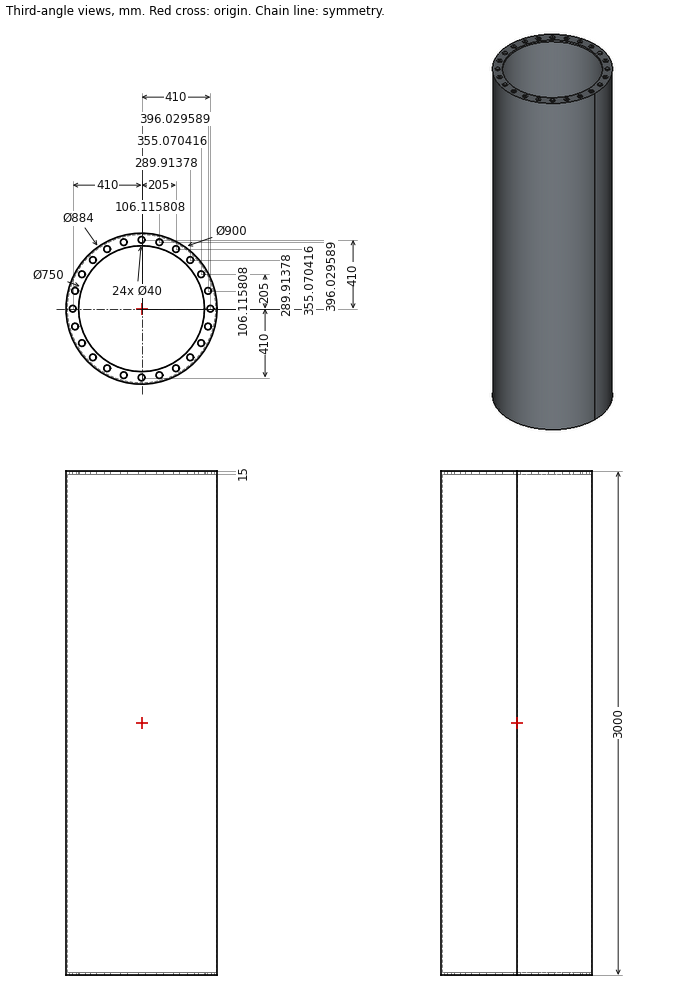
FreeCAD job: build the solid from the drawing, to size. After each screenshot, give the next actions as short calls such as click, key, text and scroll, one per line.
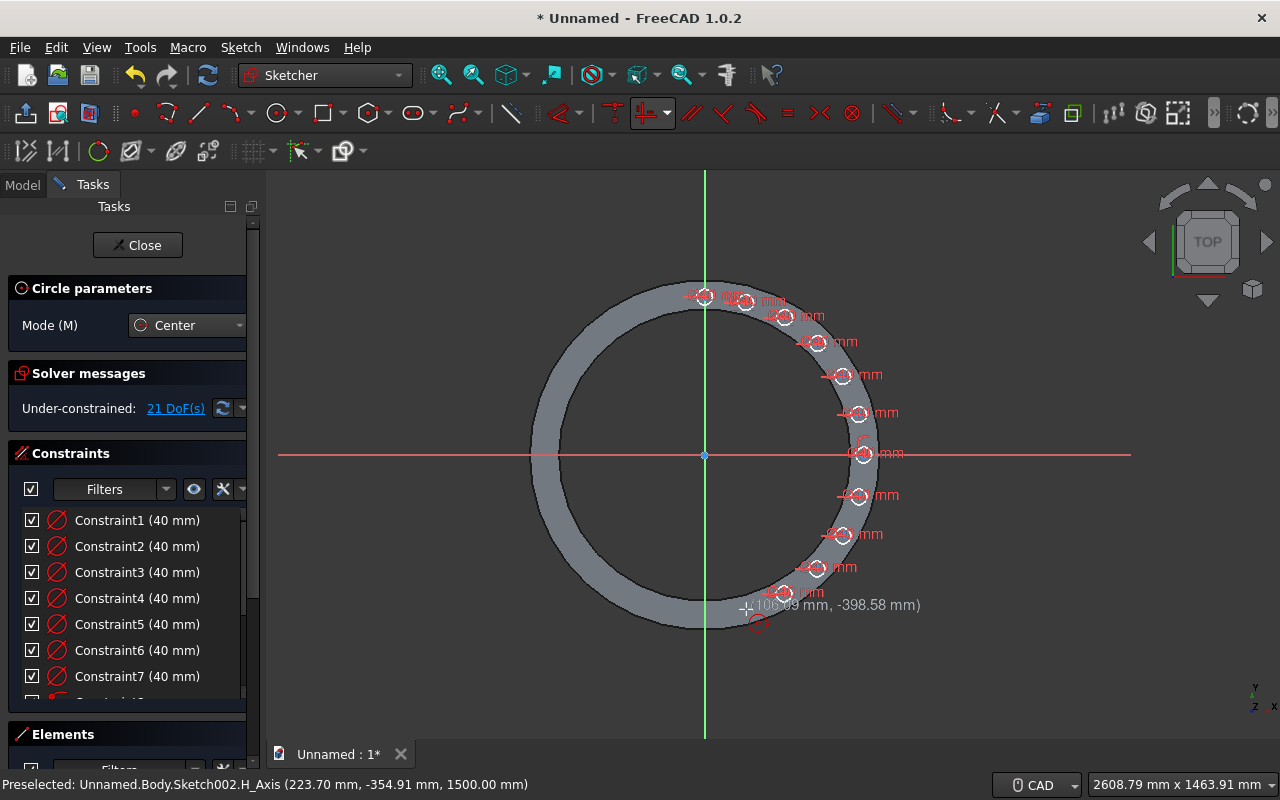
click(746, 609)
move(752, 604)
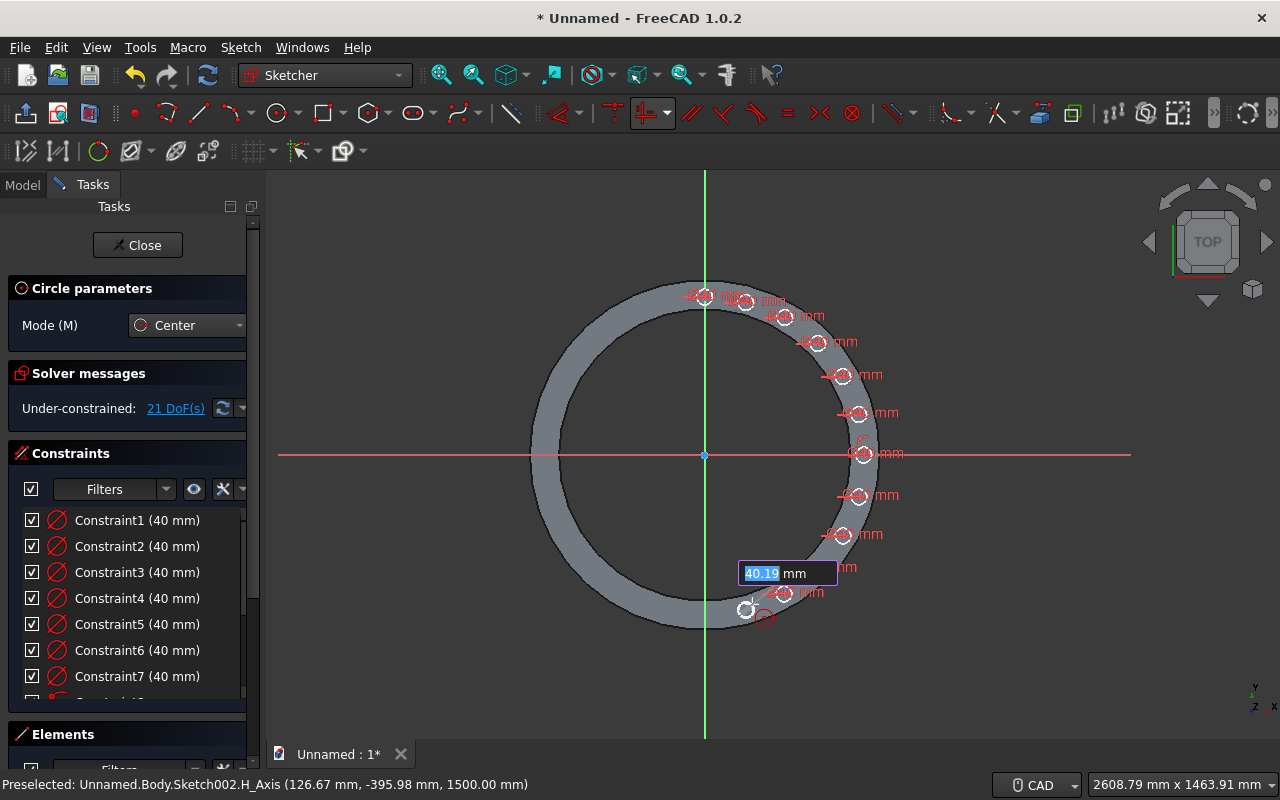
text(40)
key(Return)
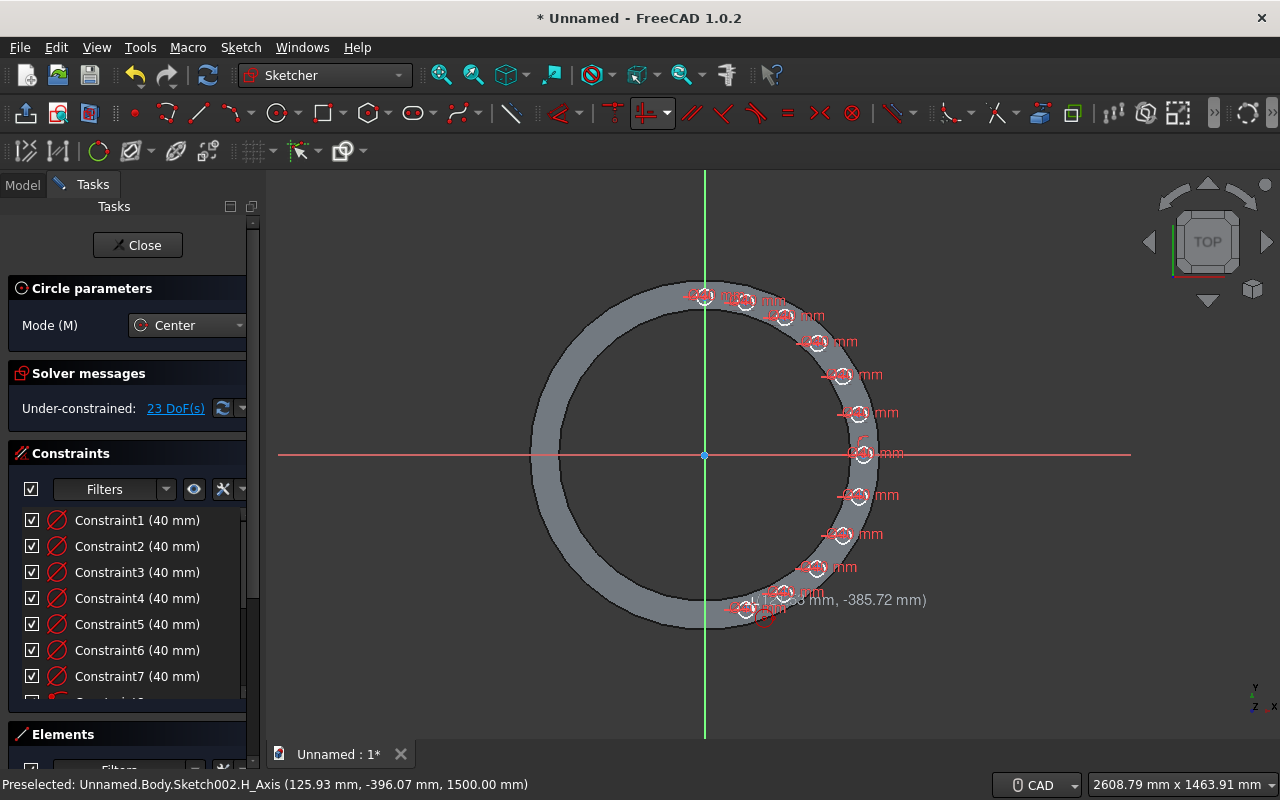
scroll(705, 614, up, 6)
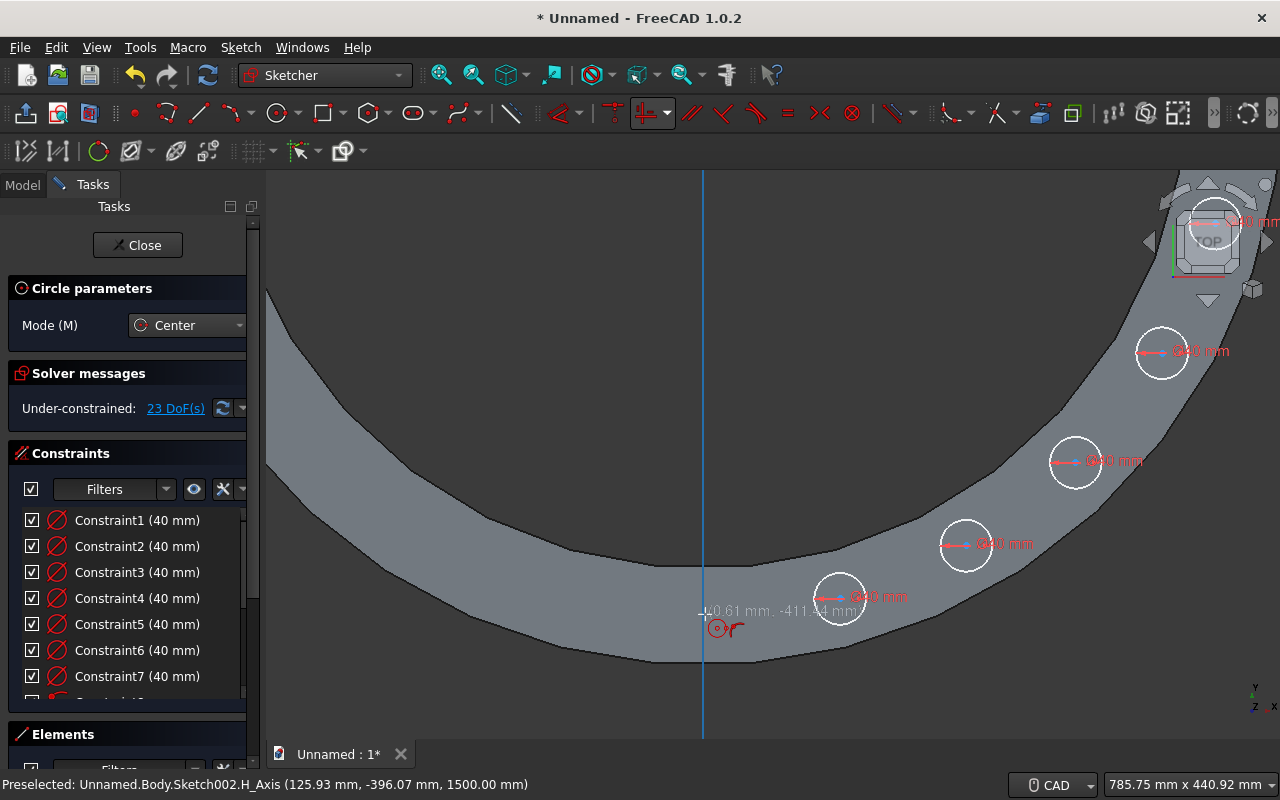
scroll(705, 614, down, 6)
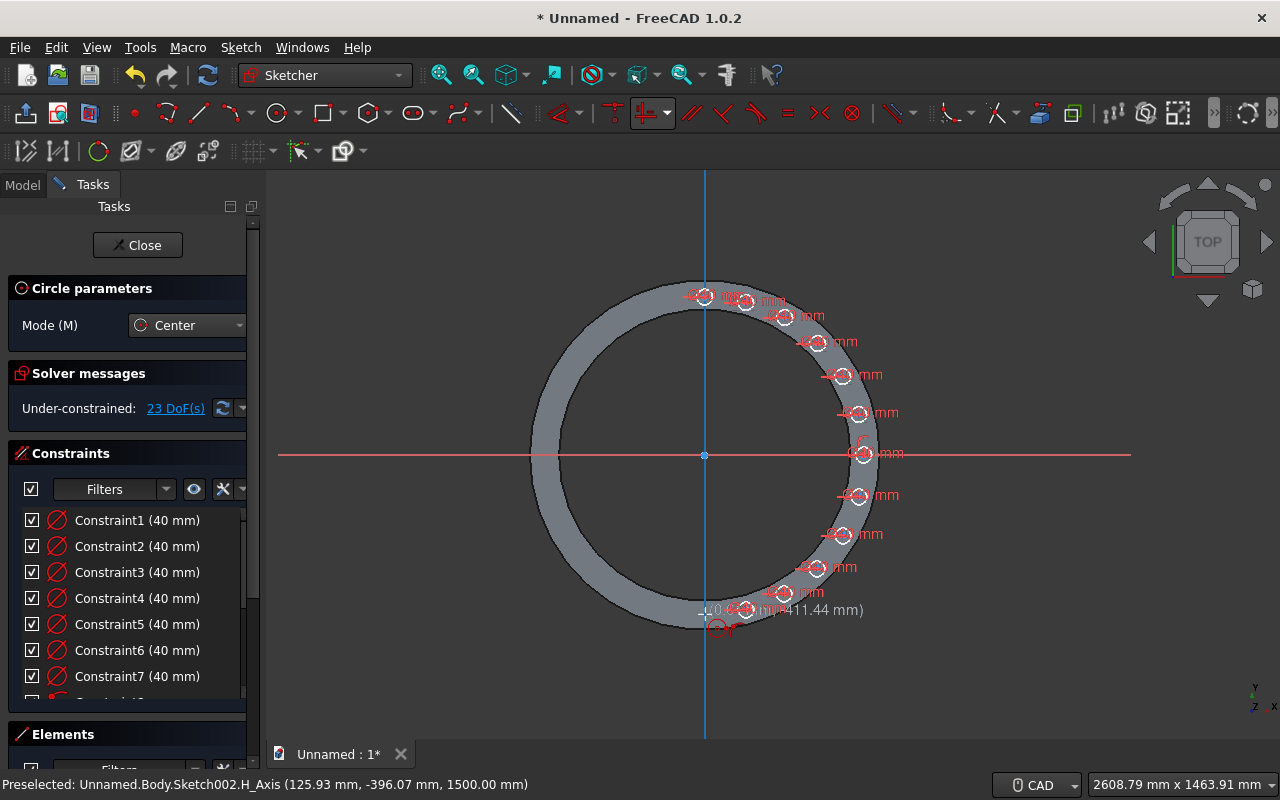
click(705, 614)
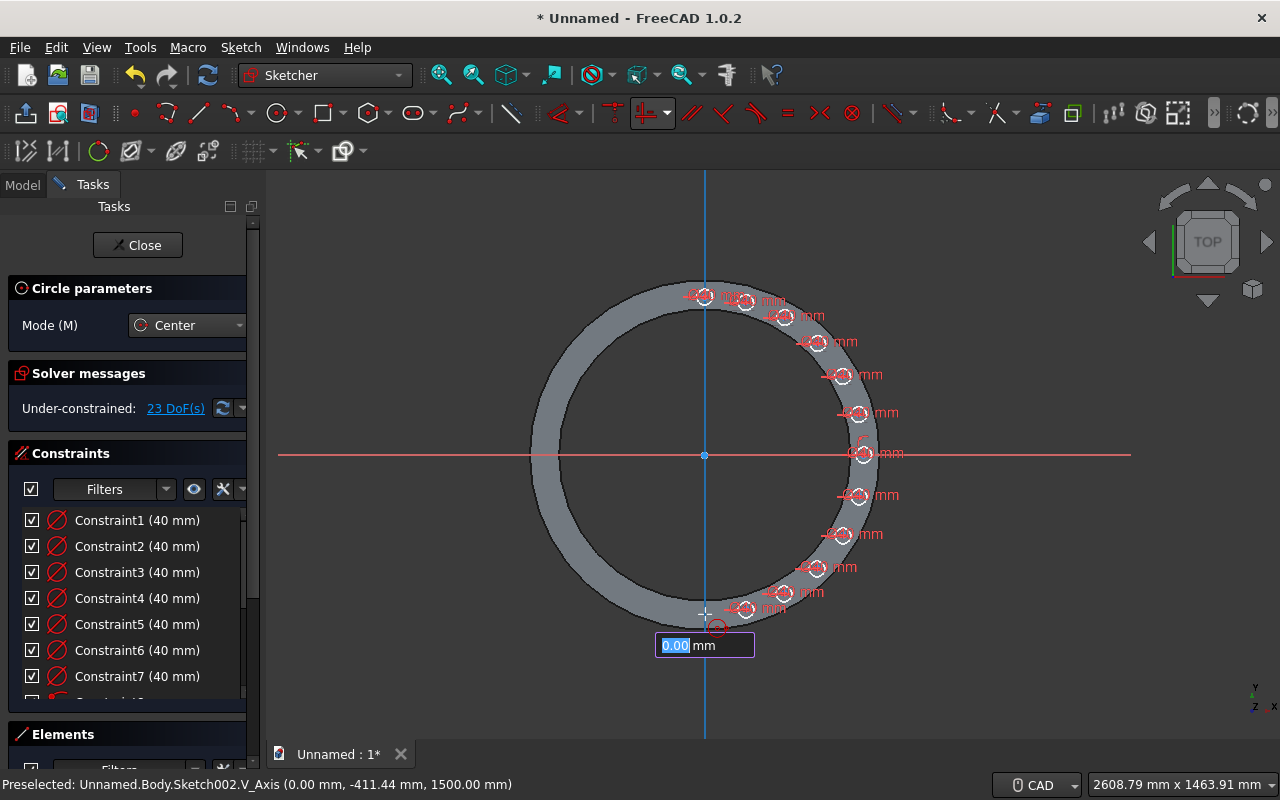
scroll(712, 612, up, 4)
move(712, 611)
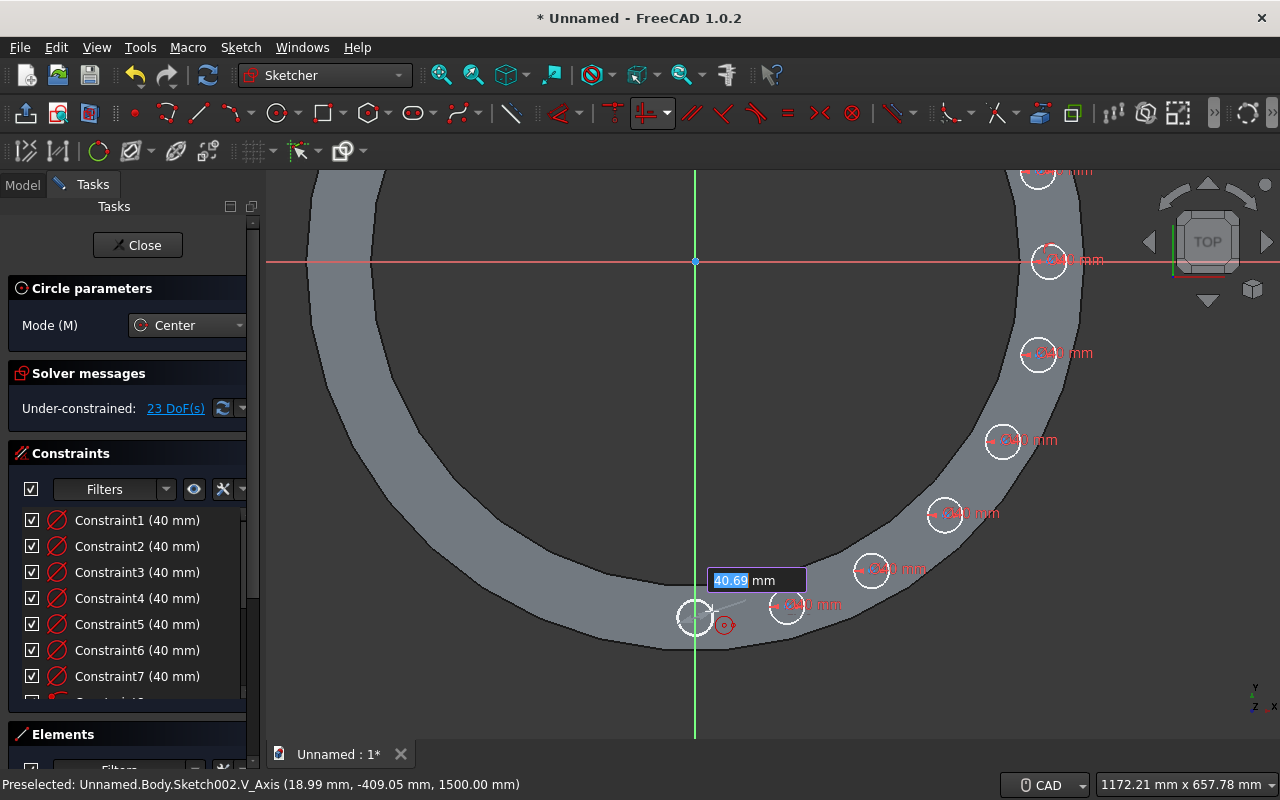
text(40)
key(Return)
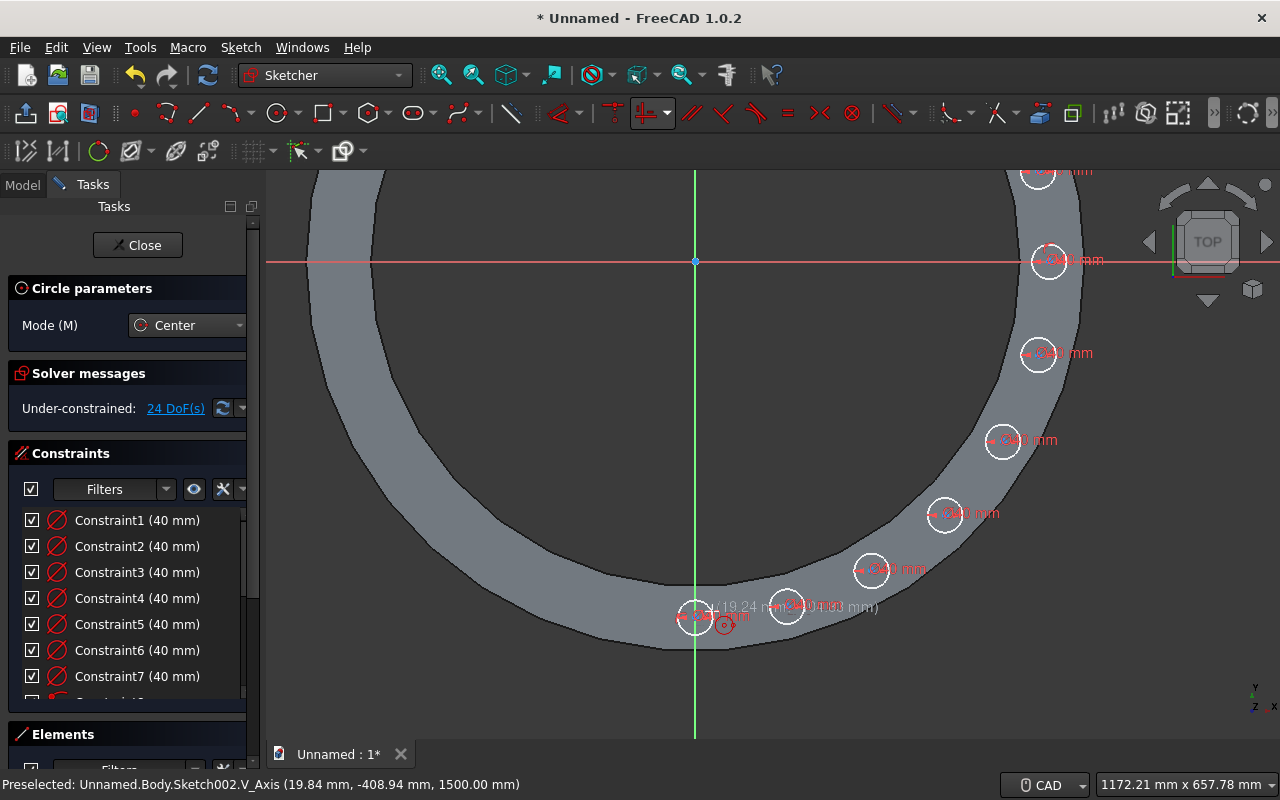
scroll(604, 604, up, 2)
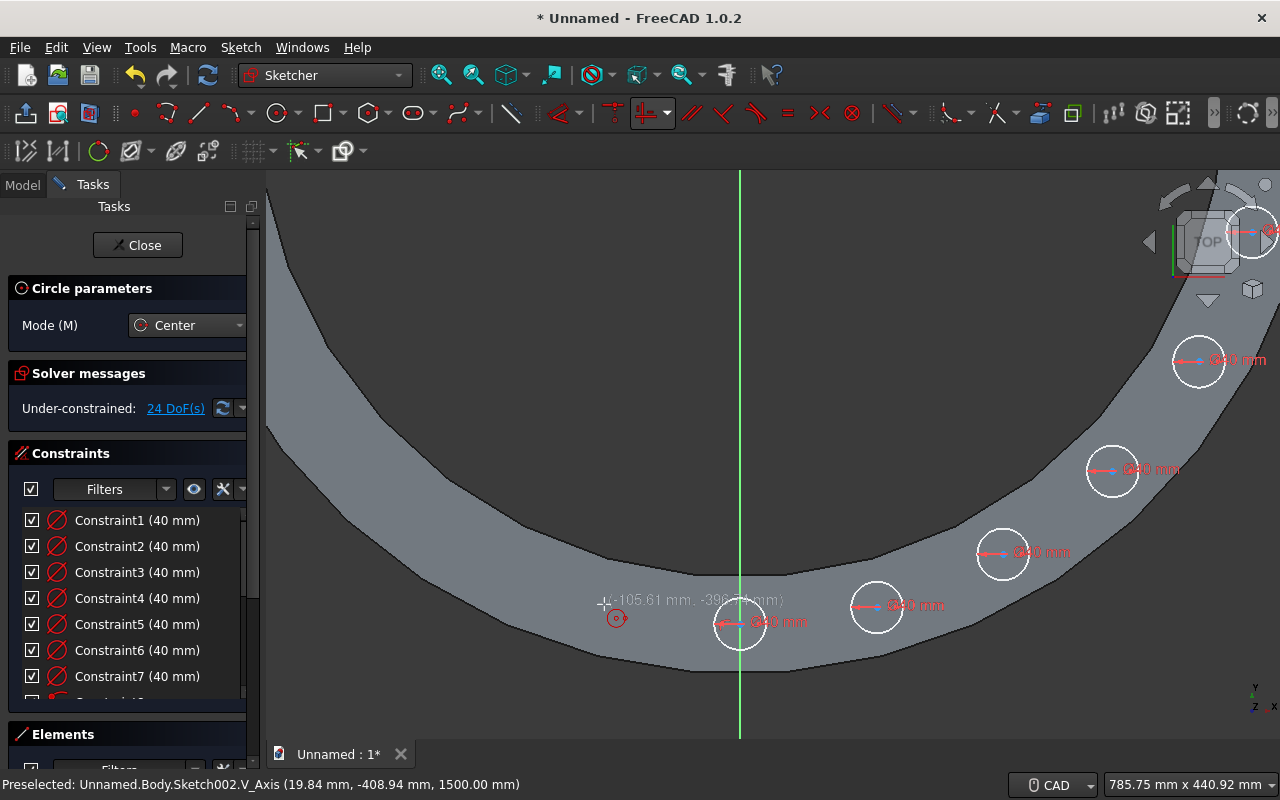
scroll(689, 610, down, 6)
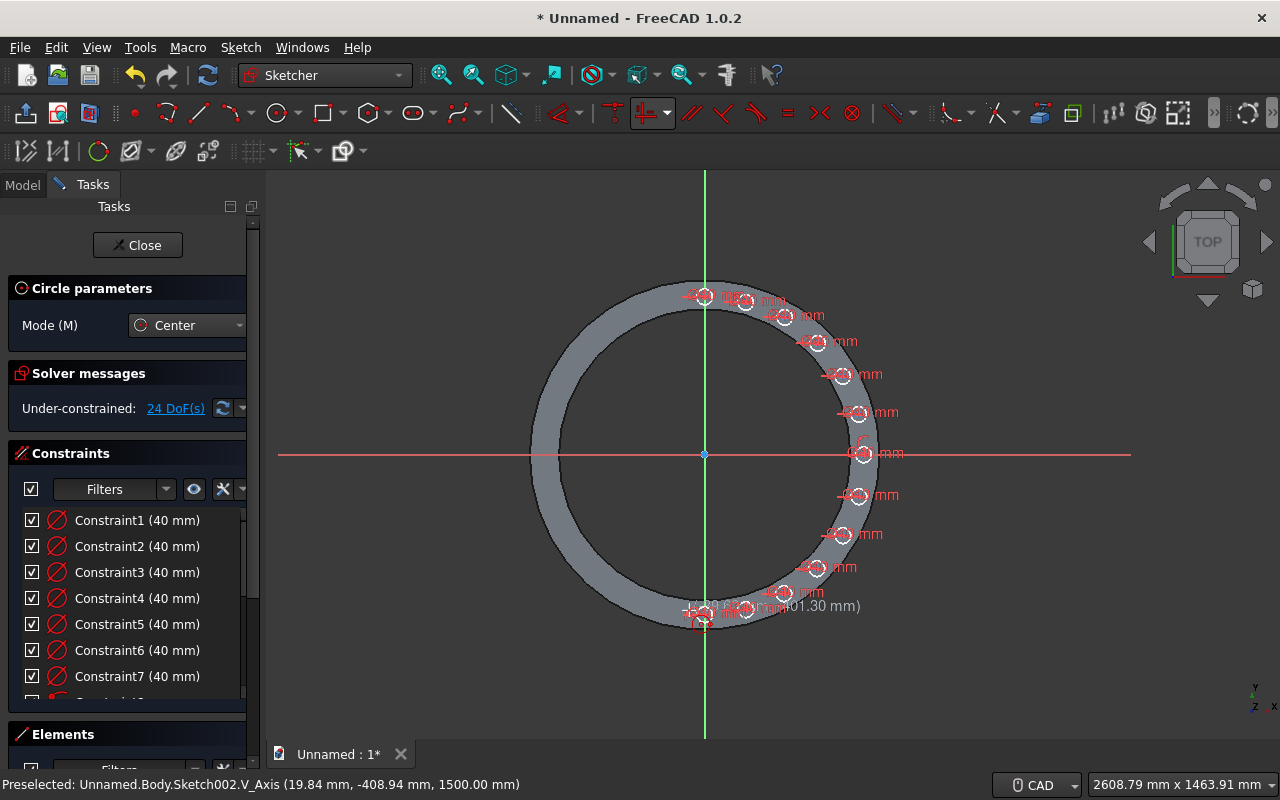
click(663, 609)
move(669, 603)